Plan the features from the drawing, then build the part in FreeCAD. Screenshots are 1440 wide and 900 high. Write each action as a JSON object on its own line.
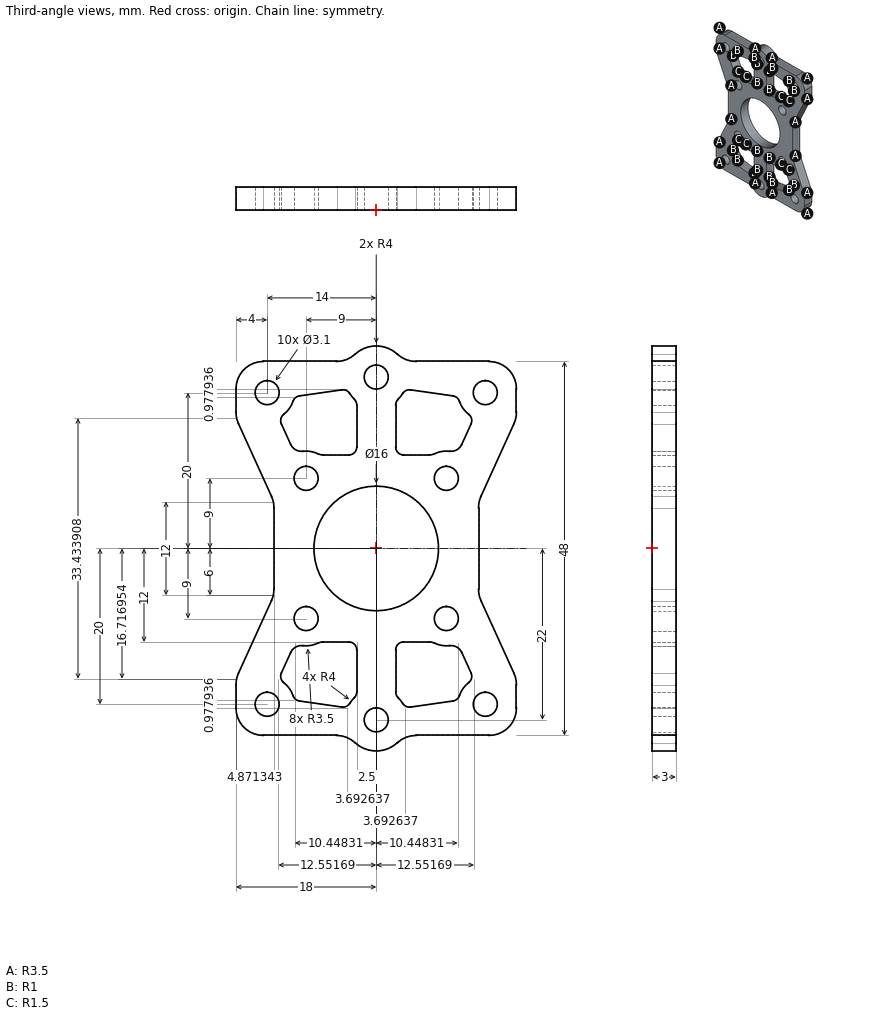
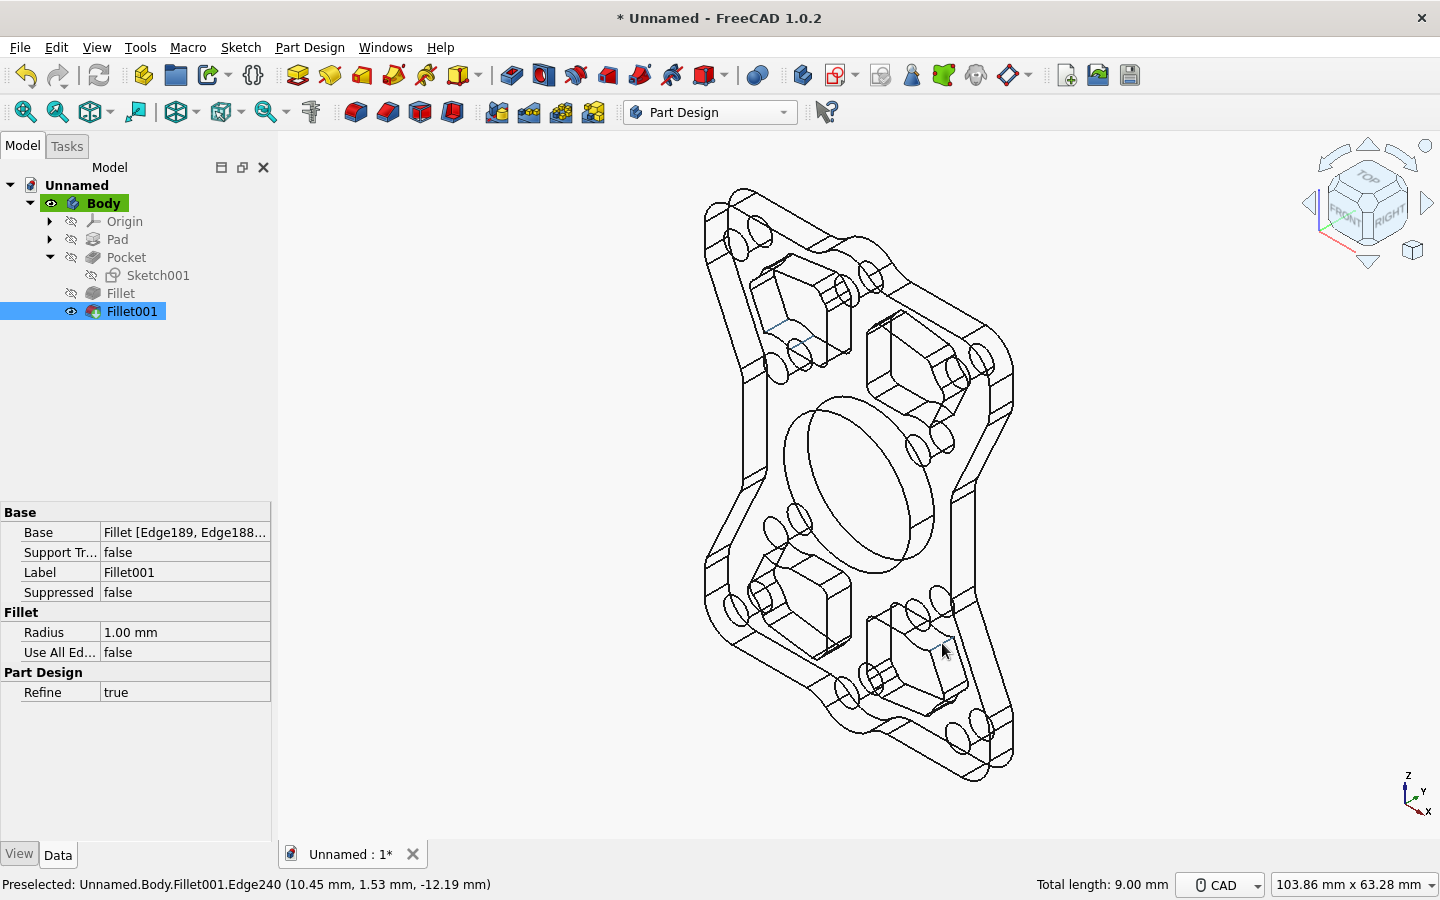
{"action": "left_click", "coordinate": [923, 622], "text": "ctrl"}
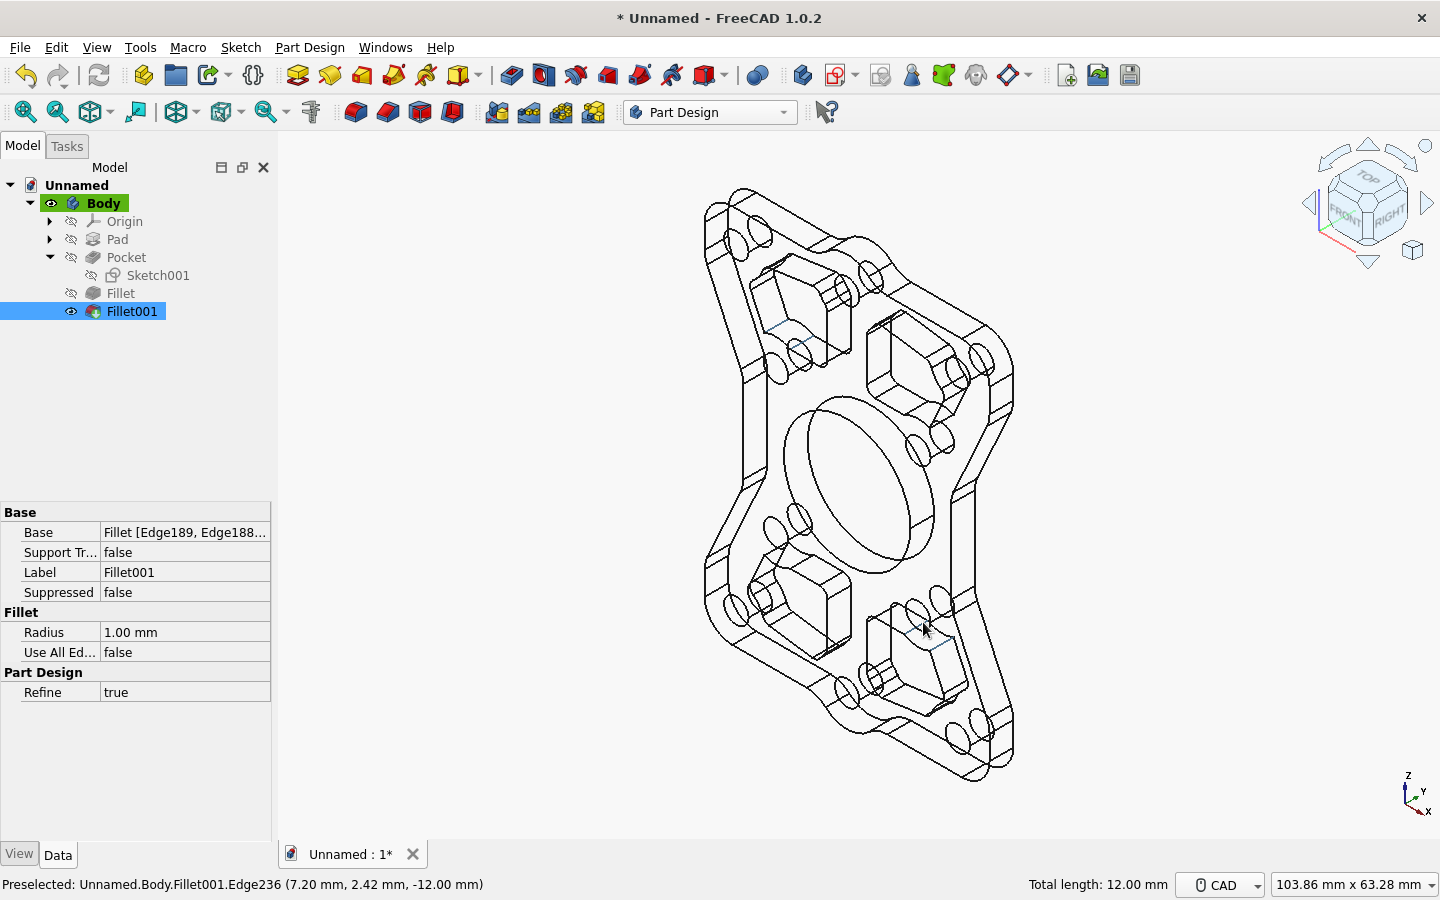
{"action": "left_click", "coordinate": [916, 407], "text": "ctrl"}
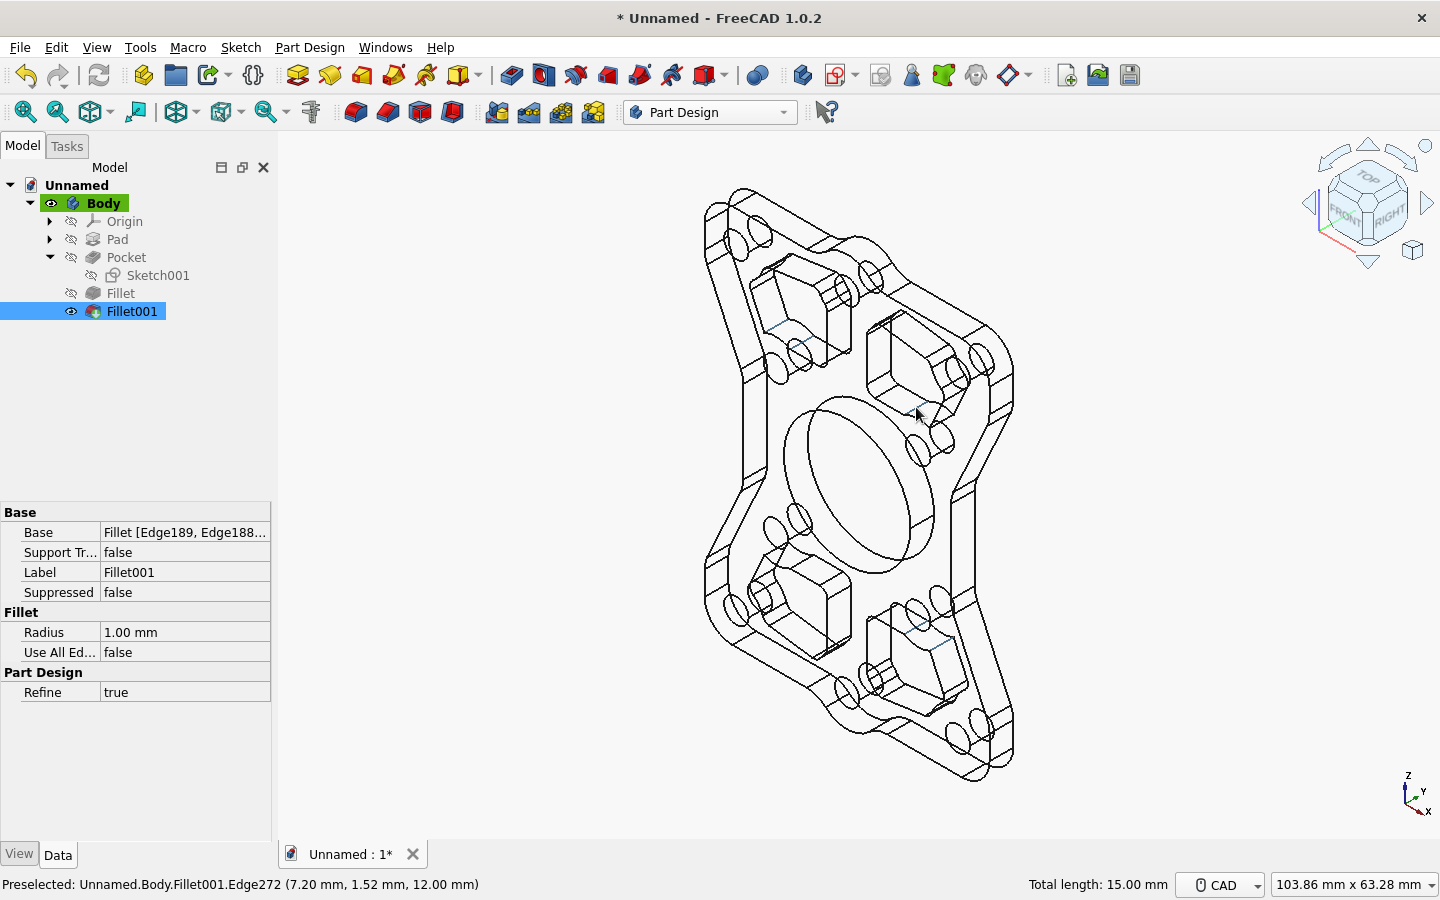
{"action": "left_click", "coordinate": [942, 420], "text": "ctrl"}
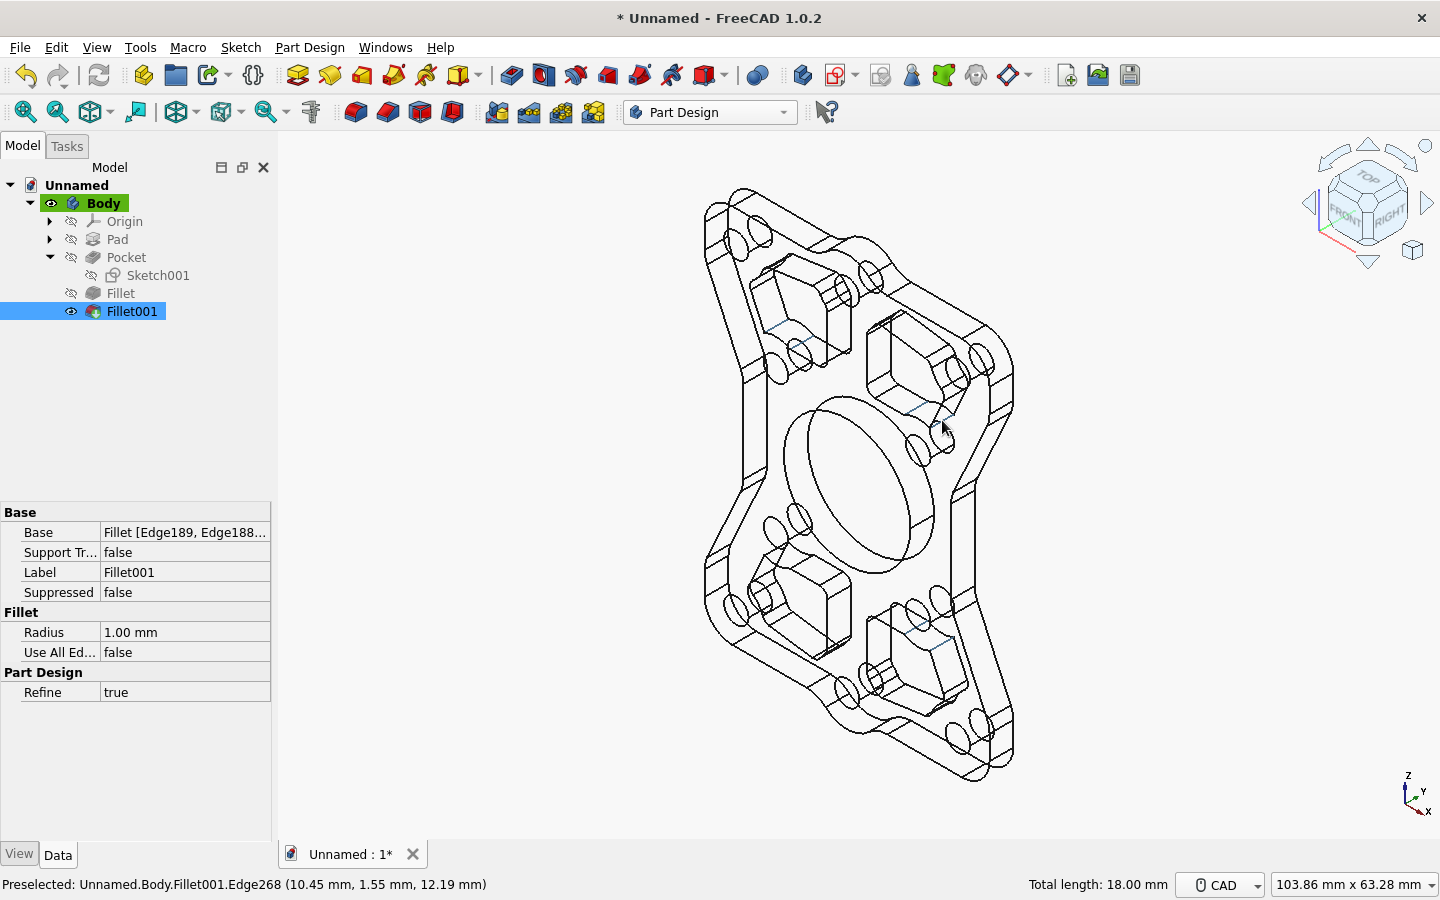
{"action": "left_click", "coordinate": [802, 561], "text": "ctrl"}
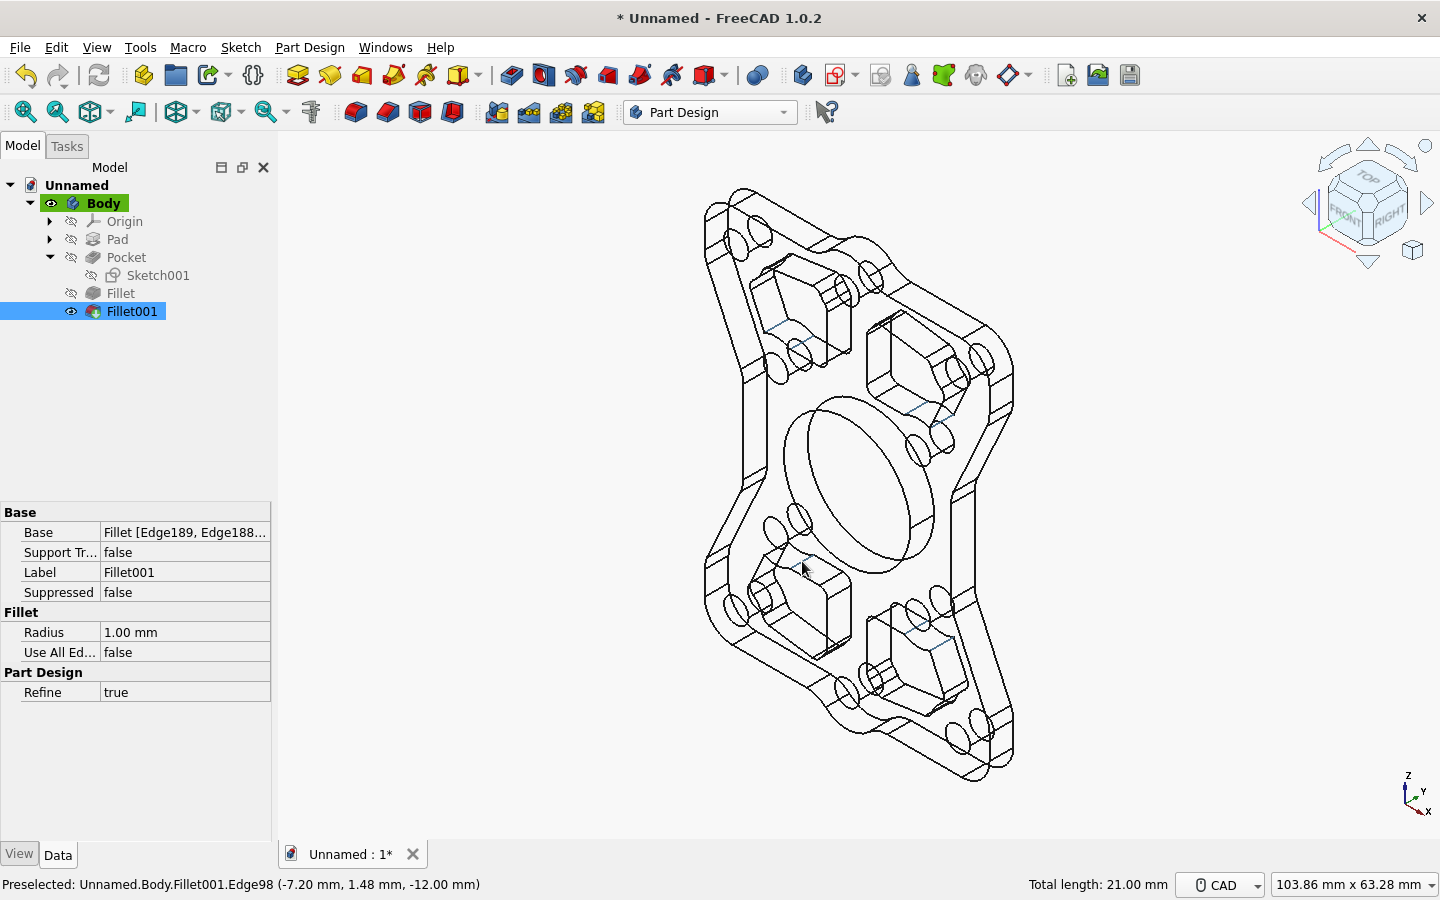
{"action": "key", "text": "2"}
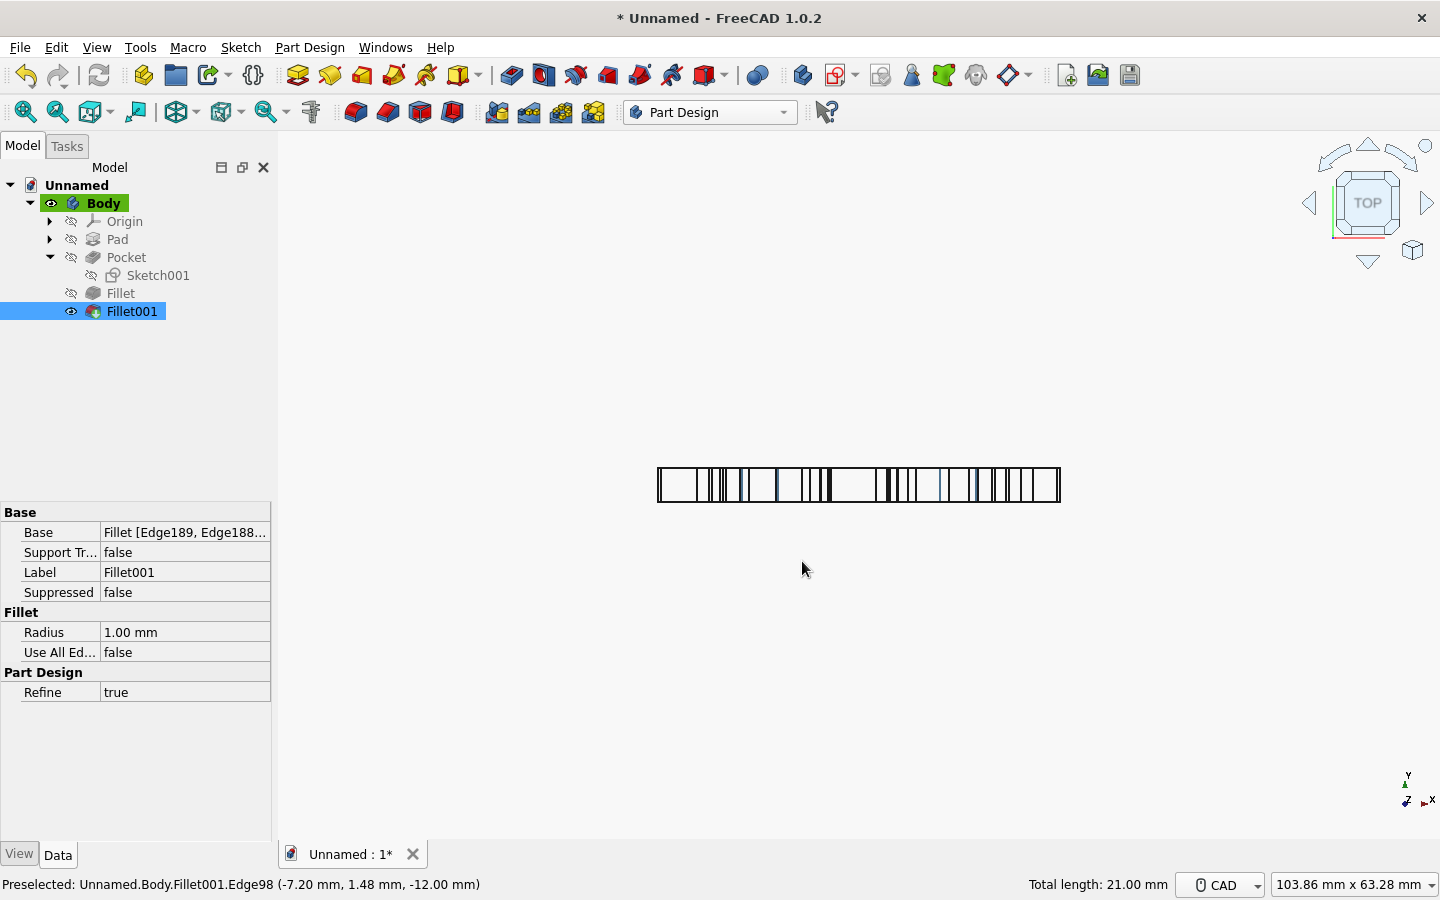
{"action": "left_click", "coordinate": [26, 112]}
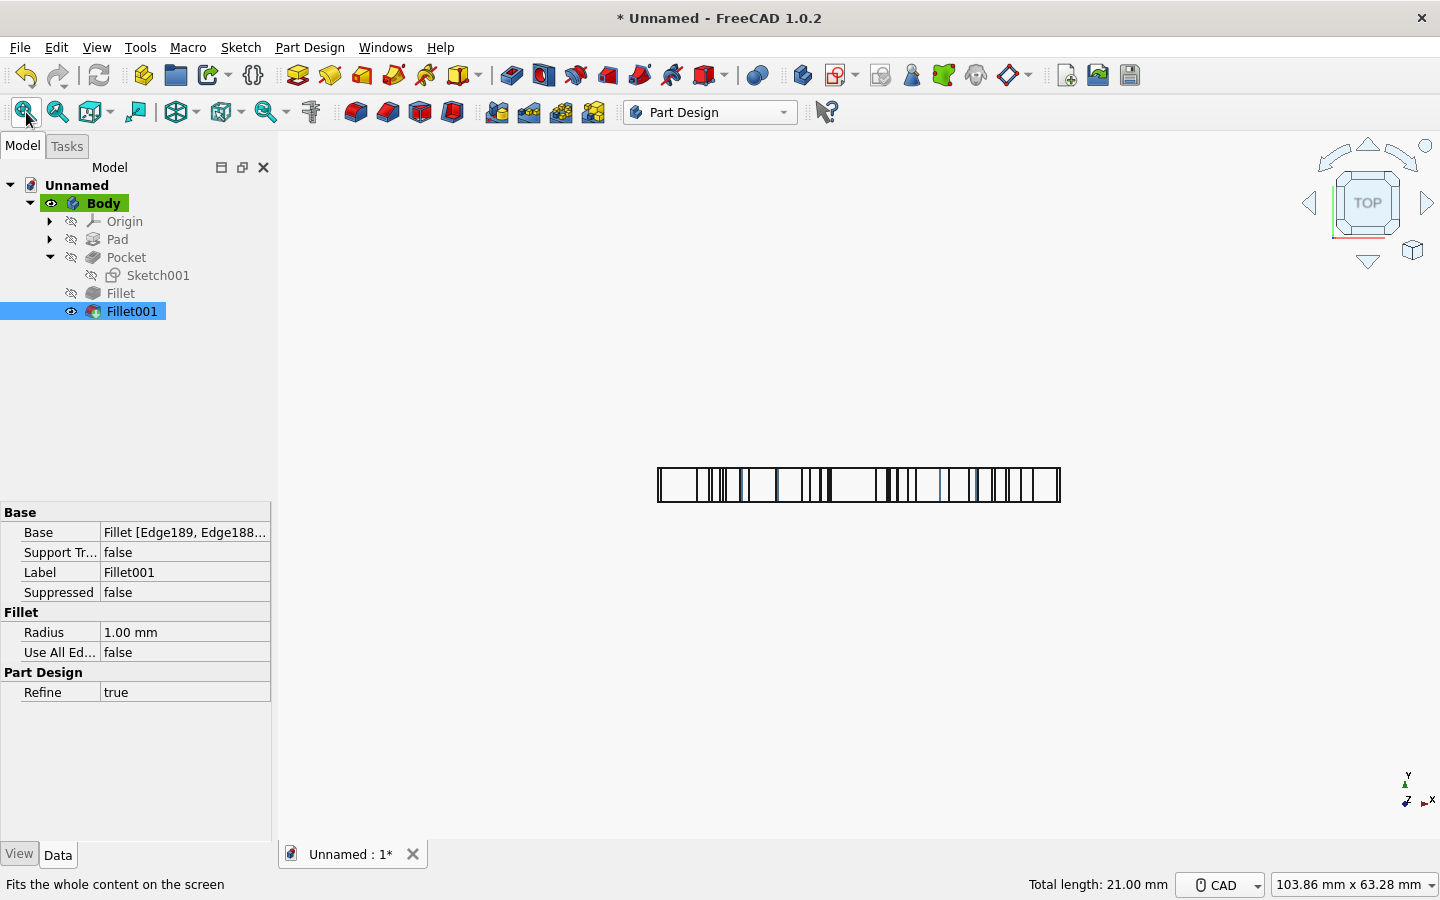
{"action": "key", "text": "1"}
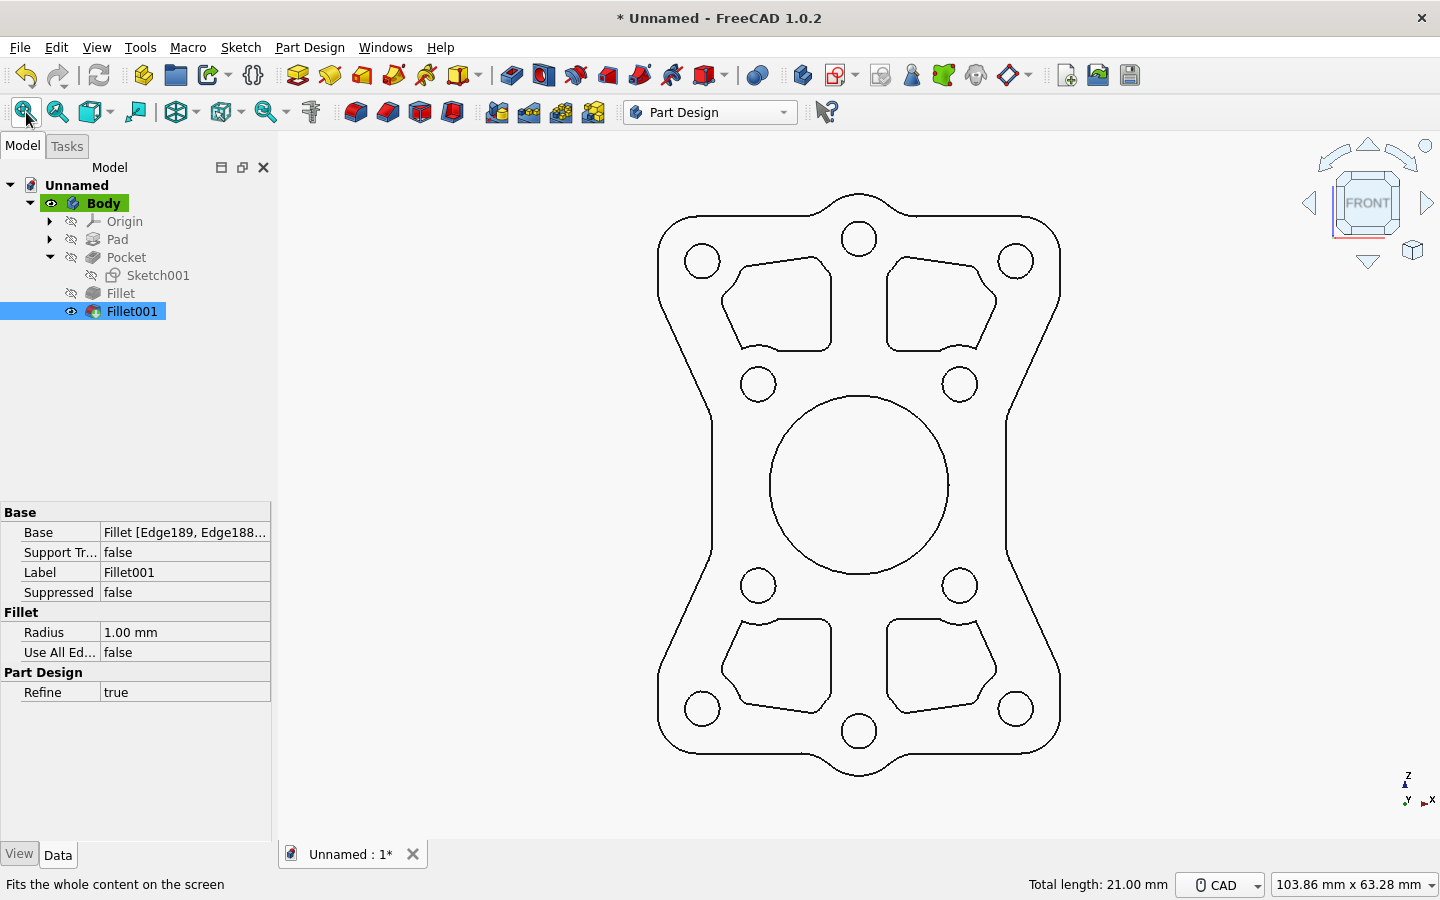
{"action": "key", "text": "3"}